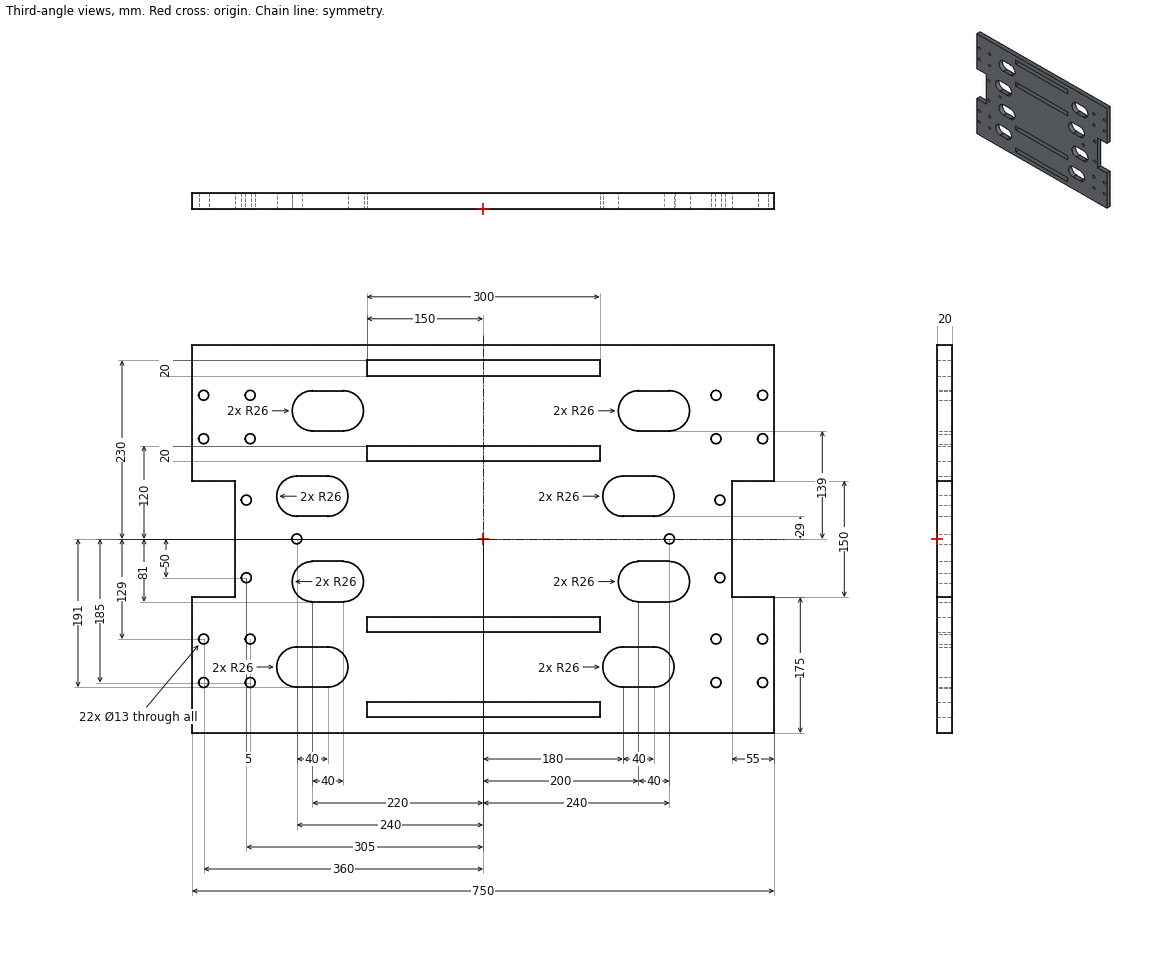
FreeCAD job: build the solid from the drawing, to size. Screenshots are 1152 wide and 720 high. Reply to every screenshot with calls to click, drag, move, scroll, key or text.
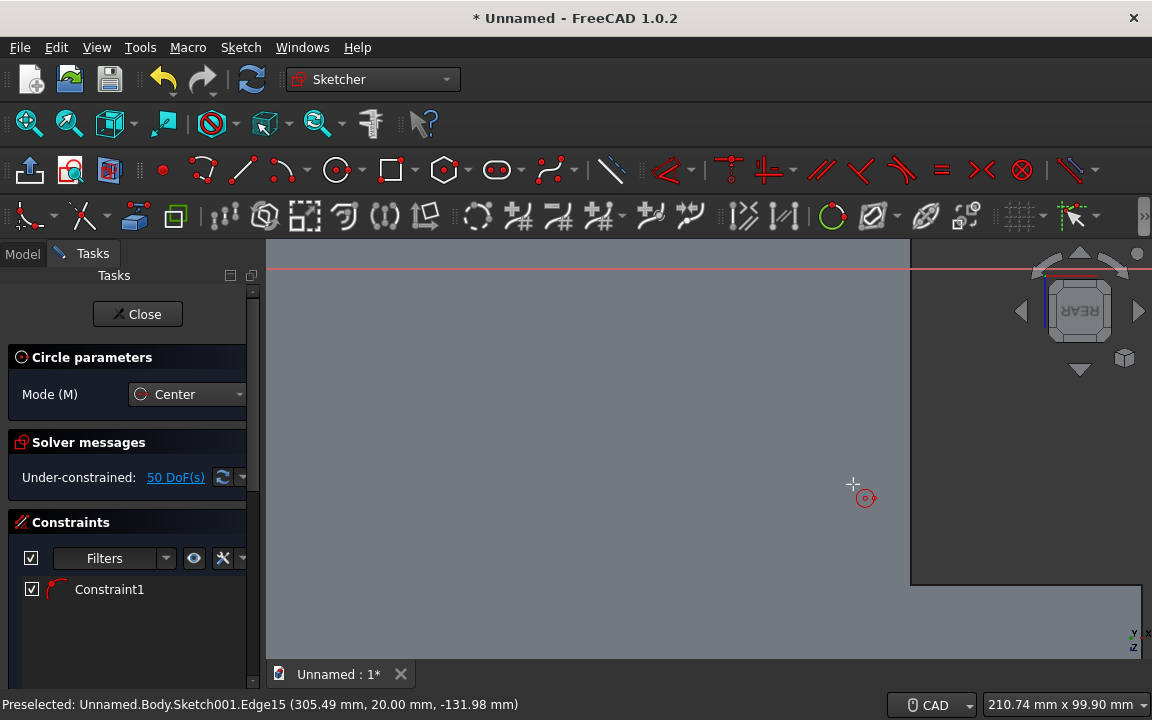
scroll(853, 485, down, 9)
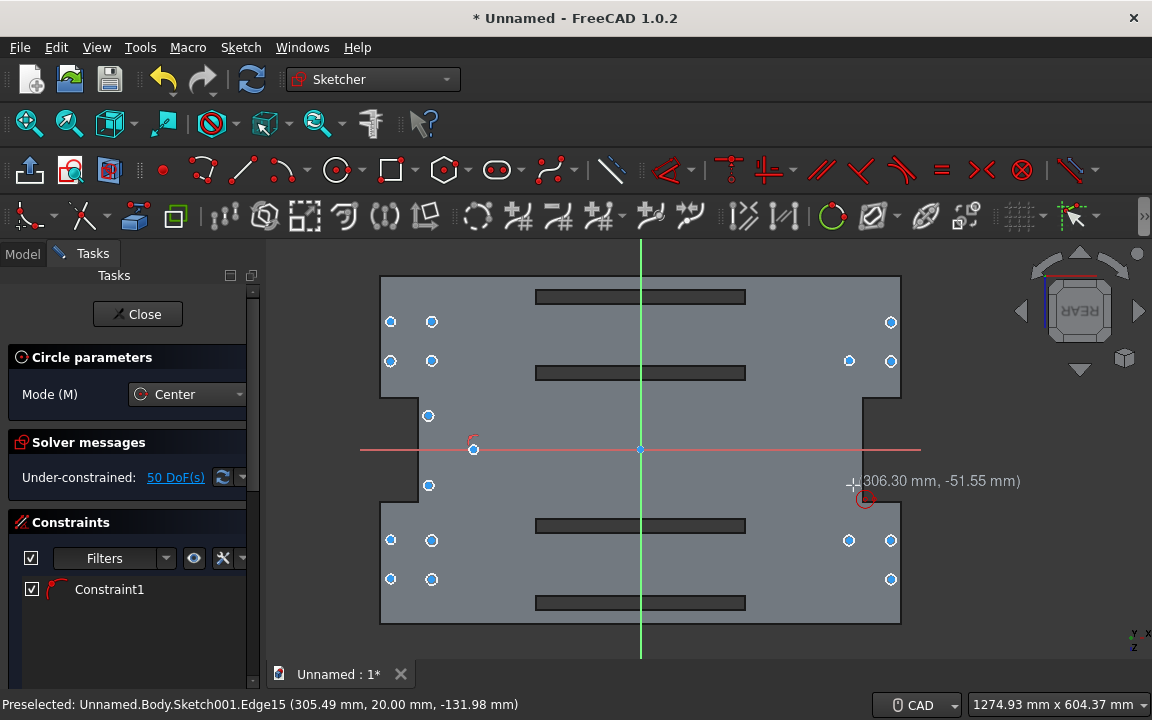
click(853, 485)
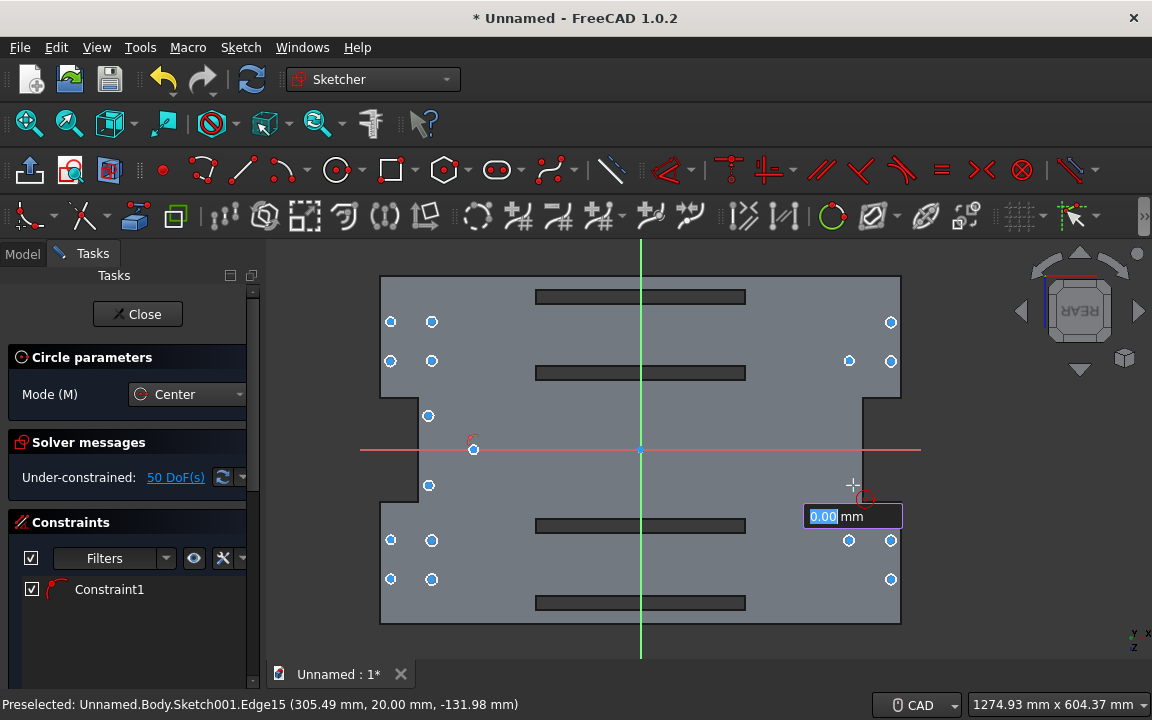
scroll(856, 481, up, 7)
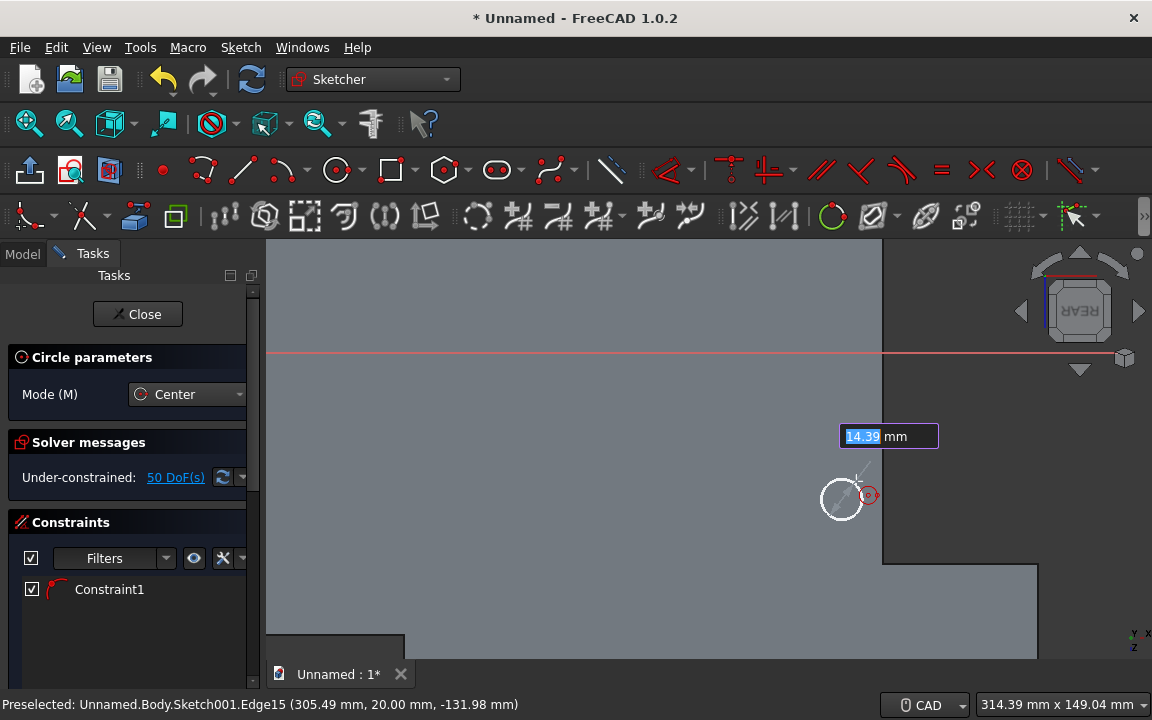
click(853, 481)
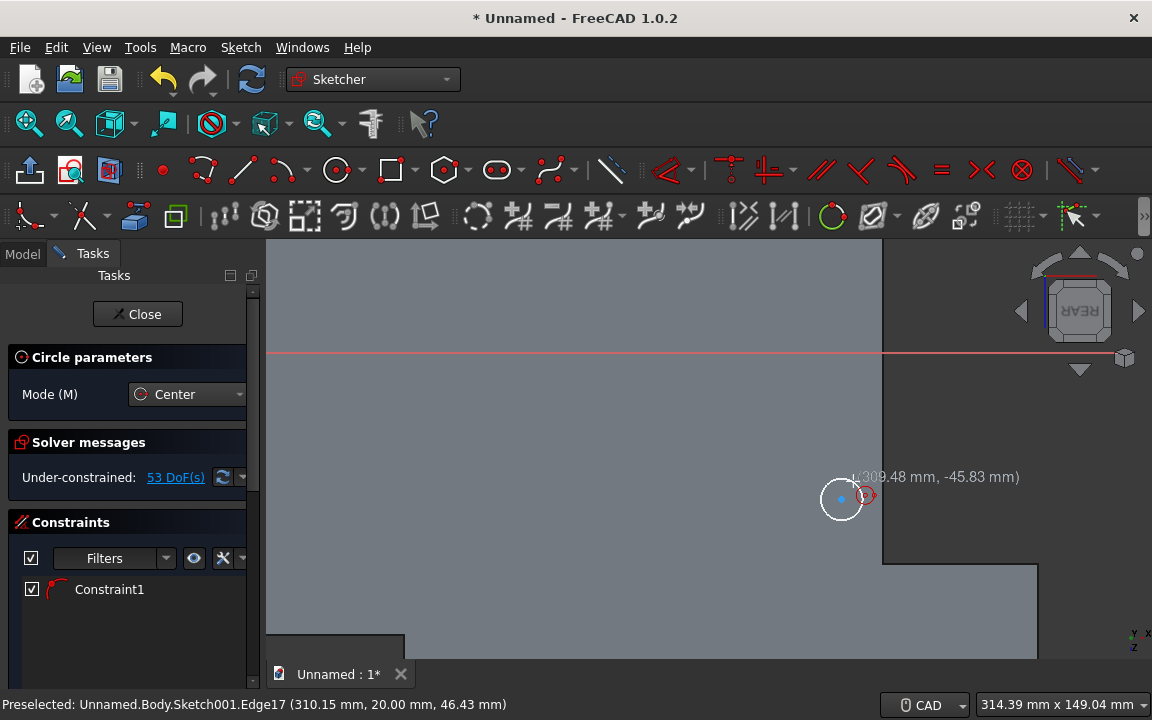
scroll(856, 480, down, 7)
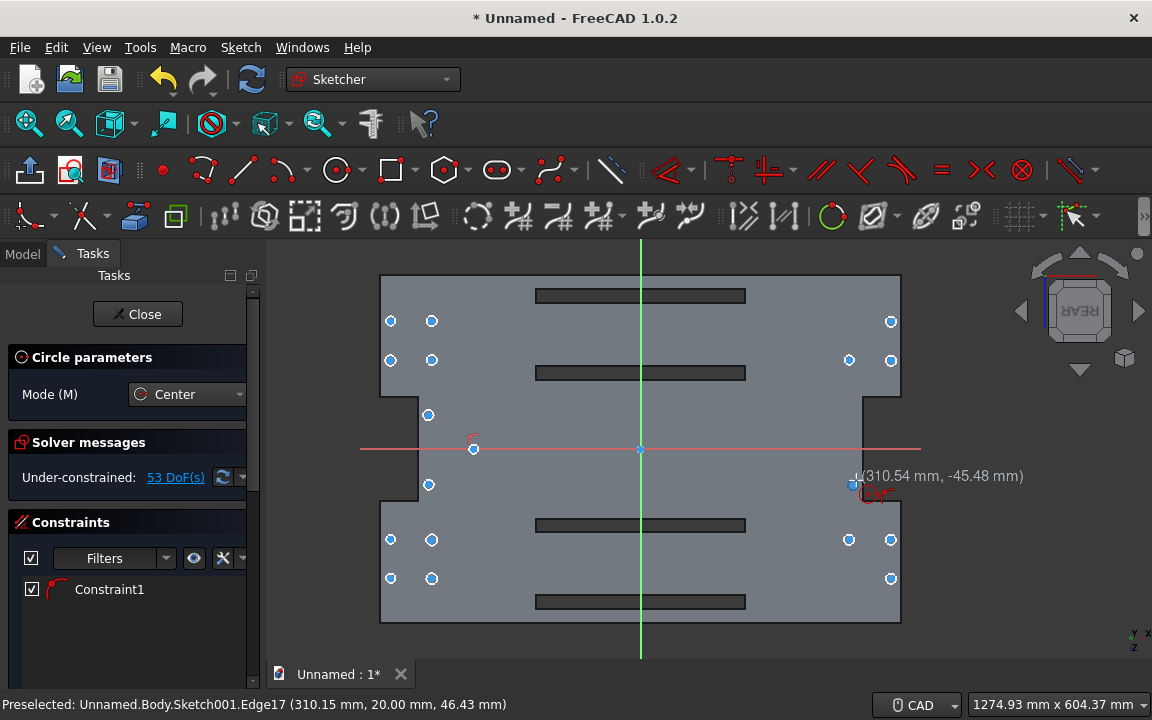
scroll(849, 578, up, 9)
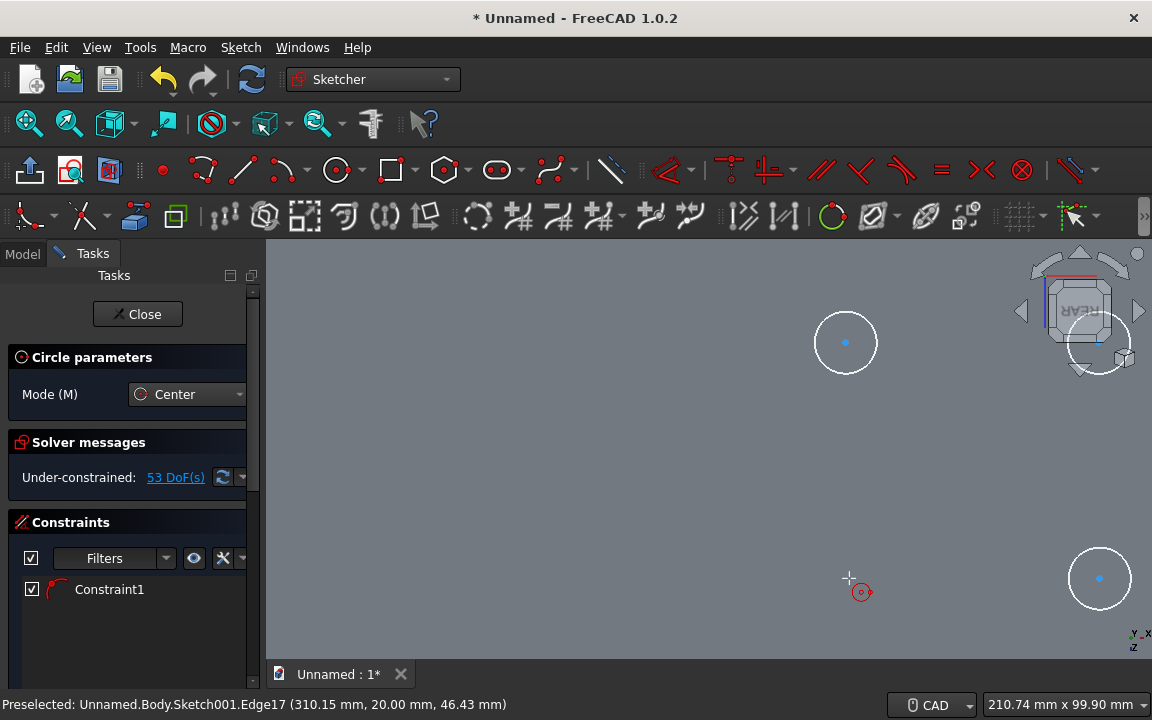
scroll(849, 579, down, 9)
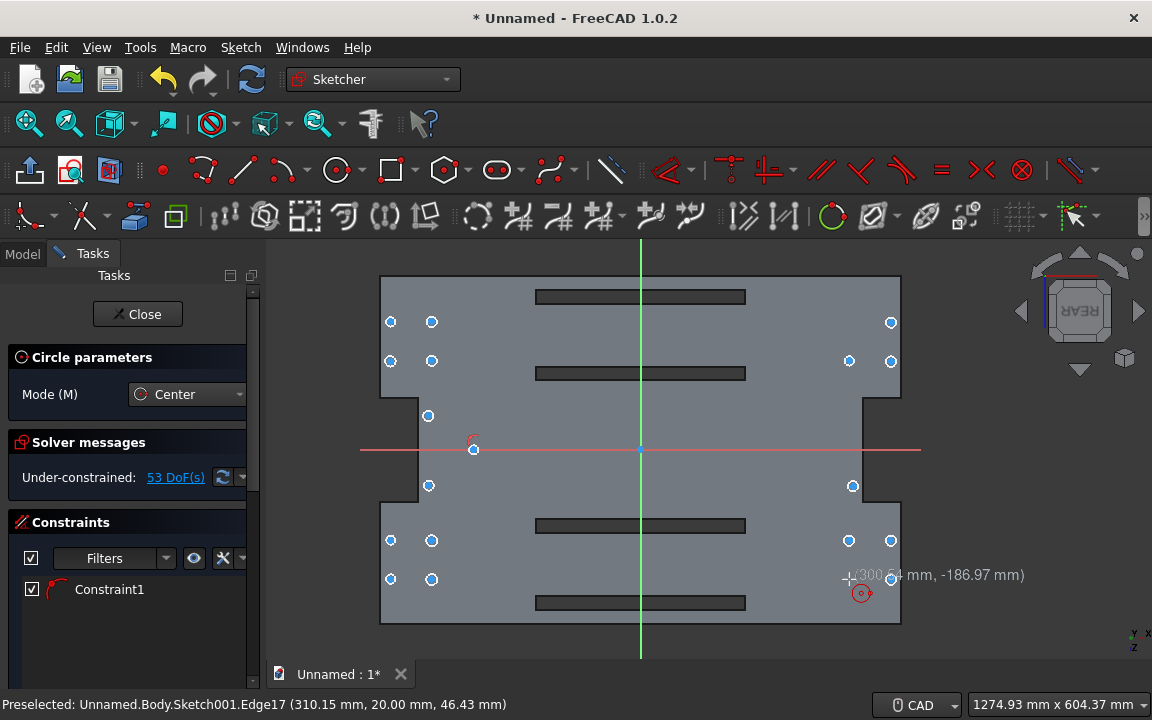
click(849, 578)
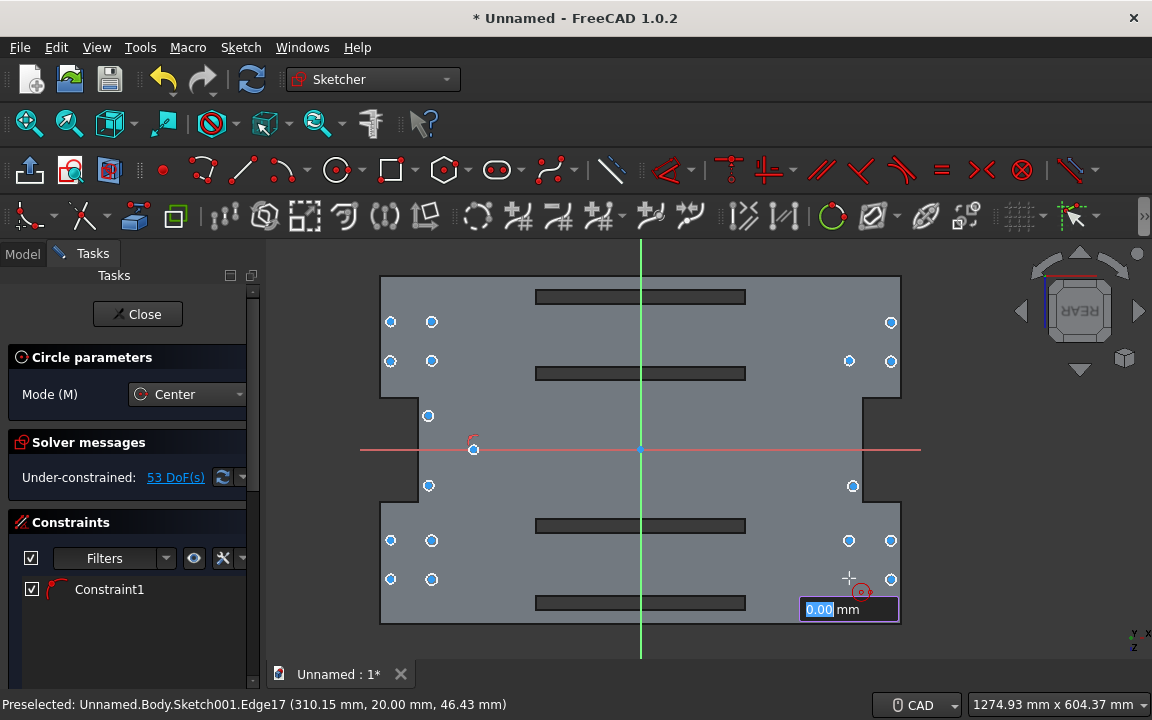
scroll(852, 575, up, 7)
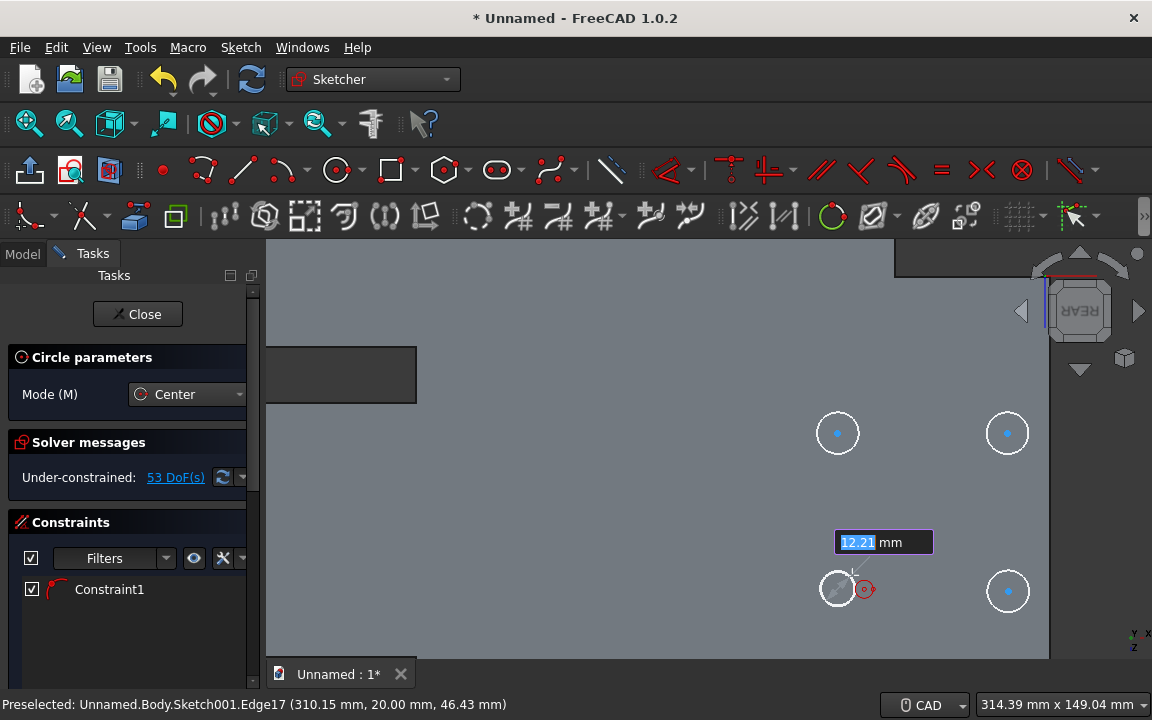
click(851, 574)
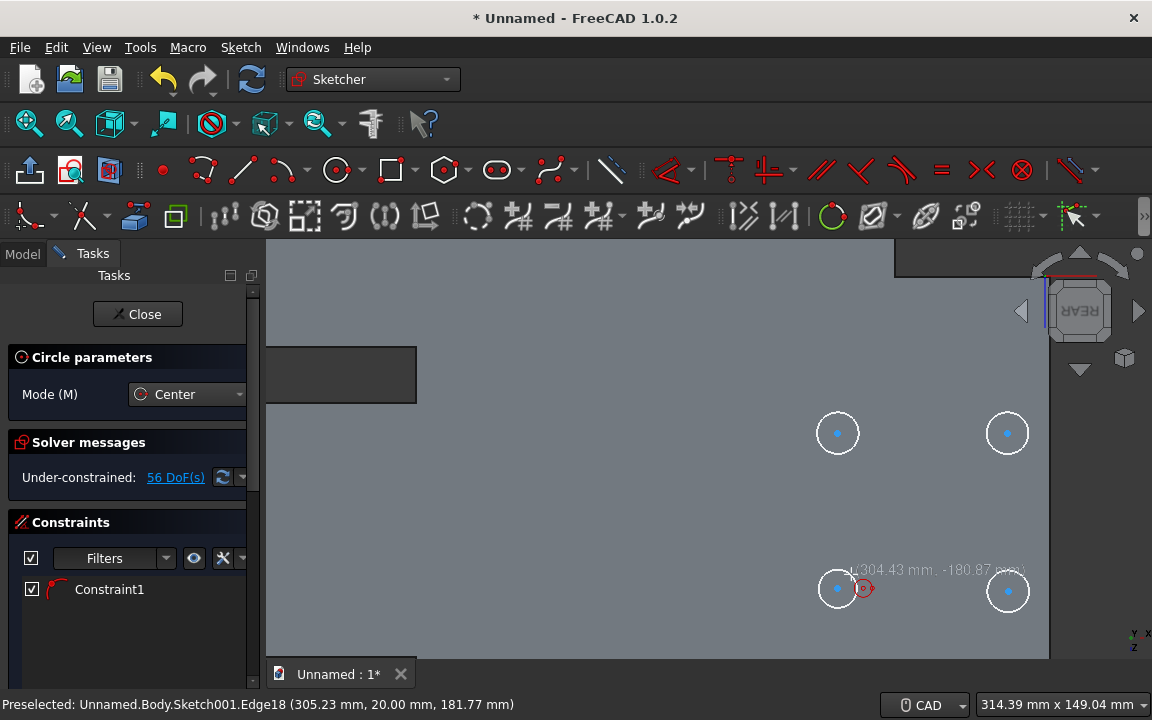
scroll(852, 575, down, 7)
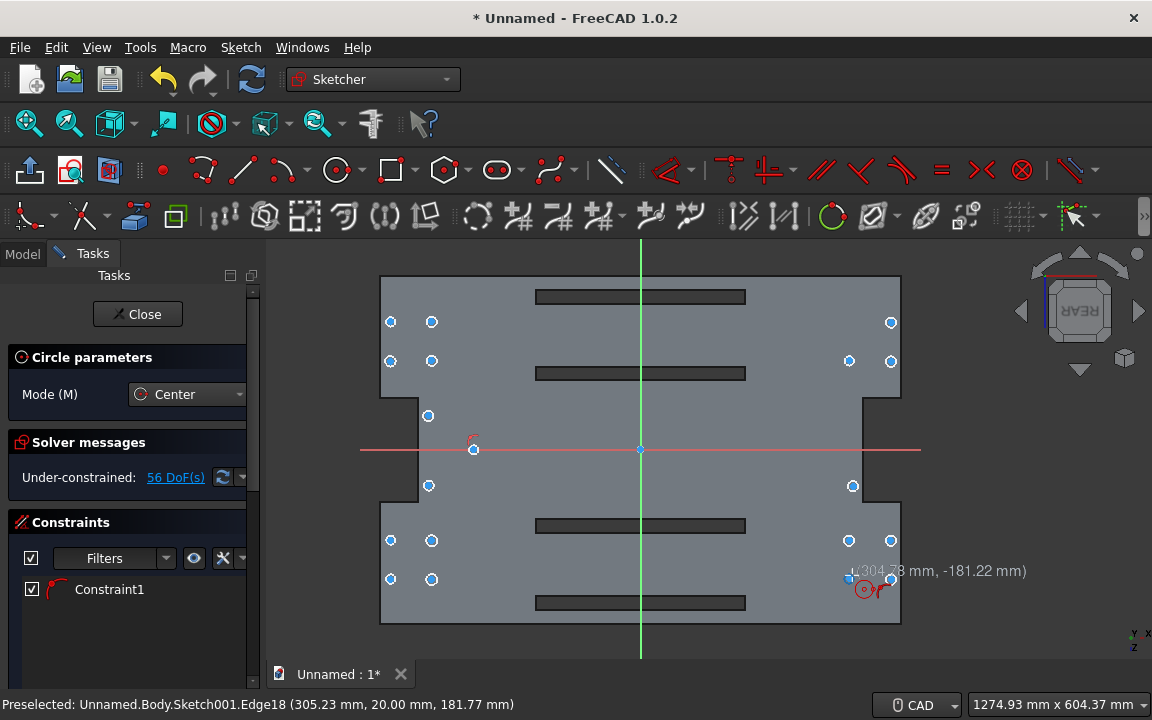
scroll(849, 321, up, 9)